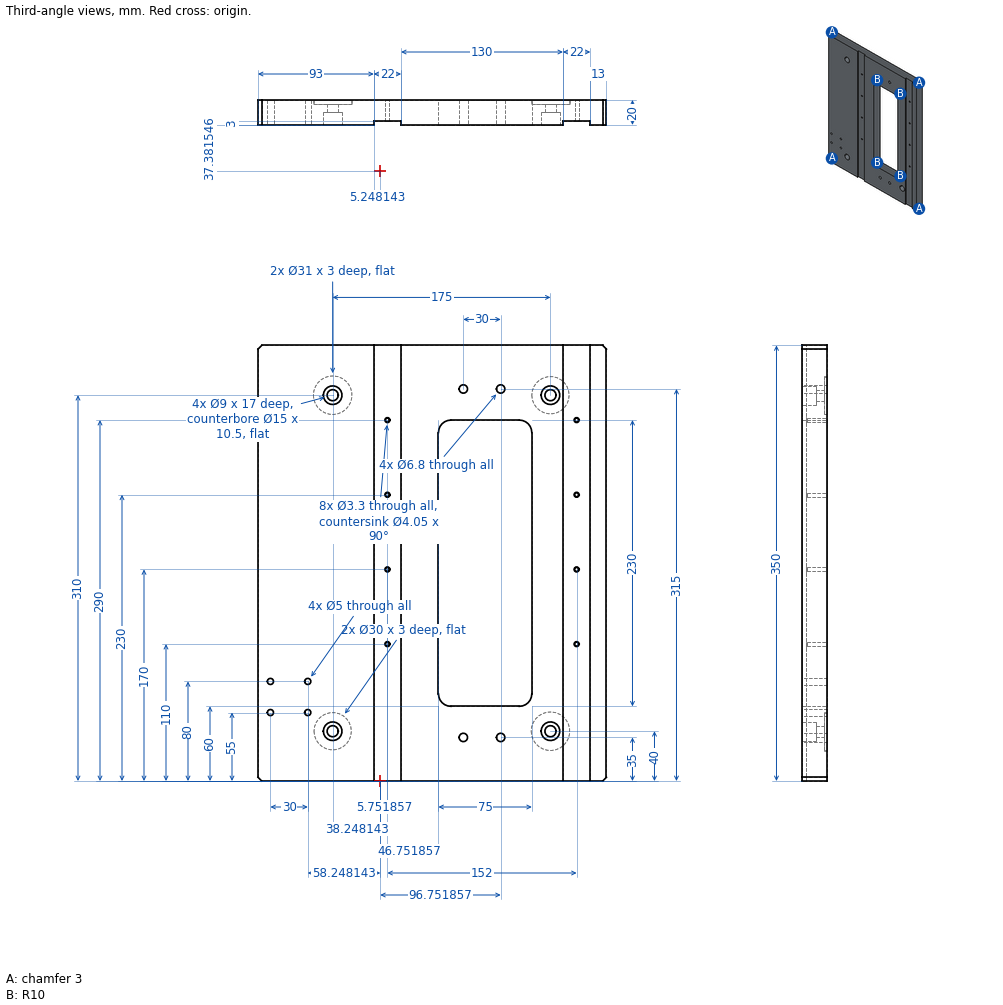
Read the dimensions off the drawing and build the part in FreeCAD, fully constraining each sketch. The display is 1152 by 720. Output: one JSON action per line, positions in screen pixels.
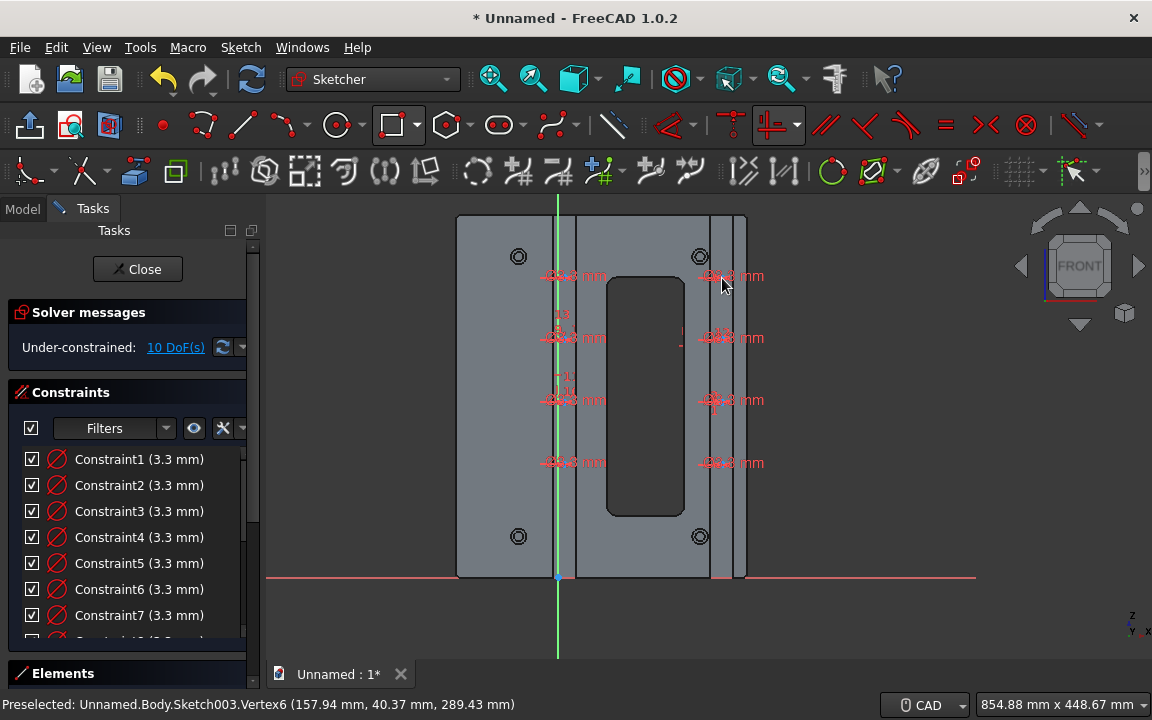
{"action": "left_click", "coordinate": [564, 278]}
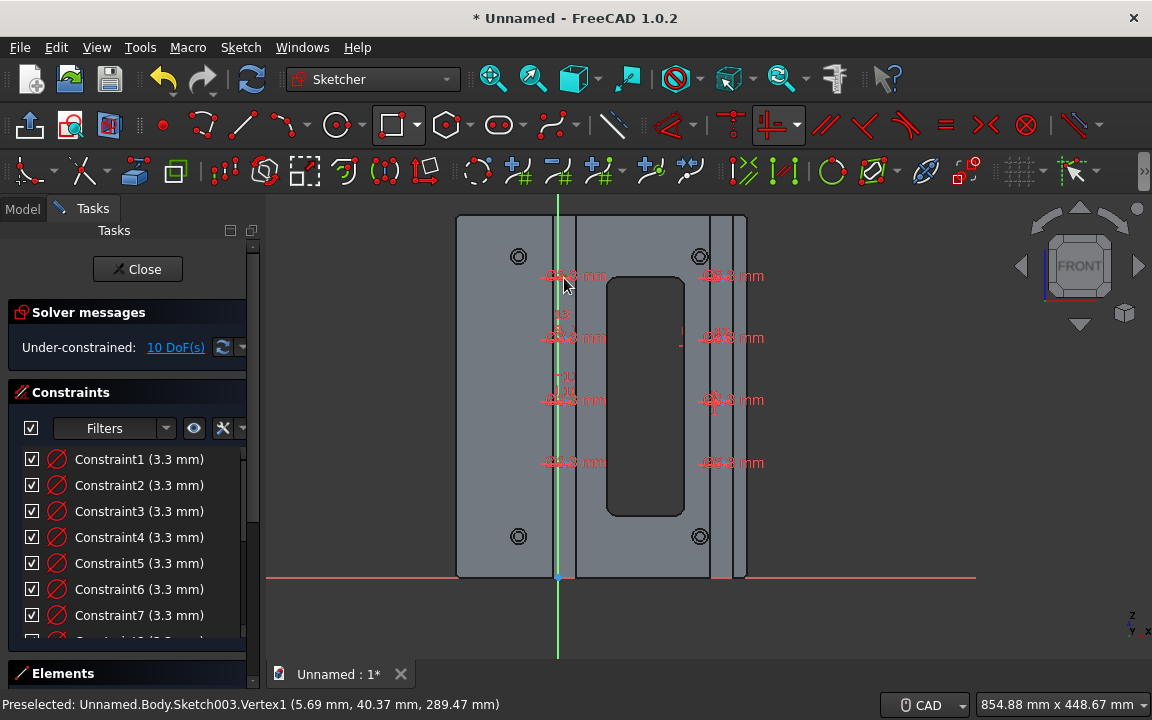
{"action": "left_click", "coordinate": [722, 278]}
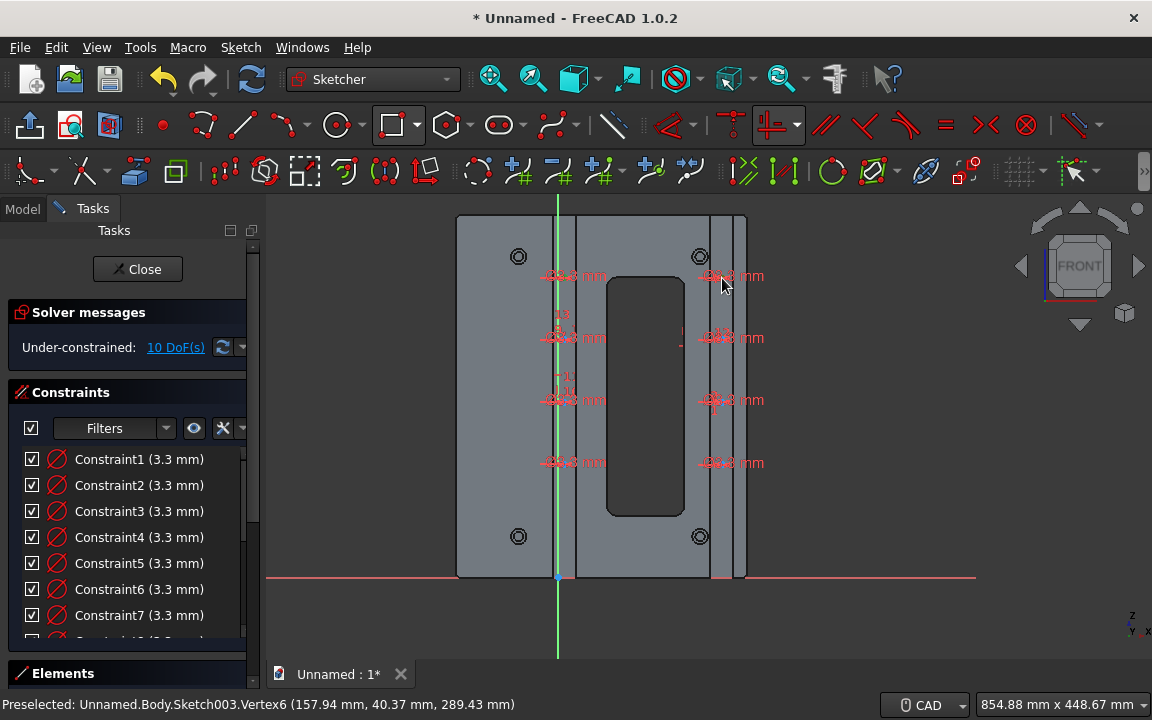
{"action": "left_click", "coordinate": [800, 126]}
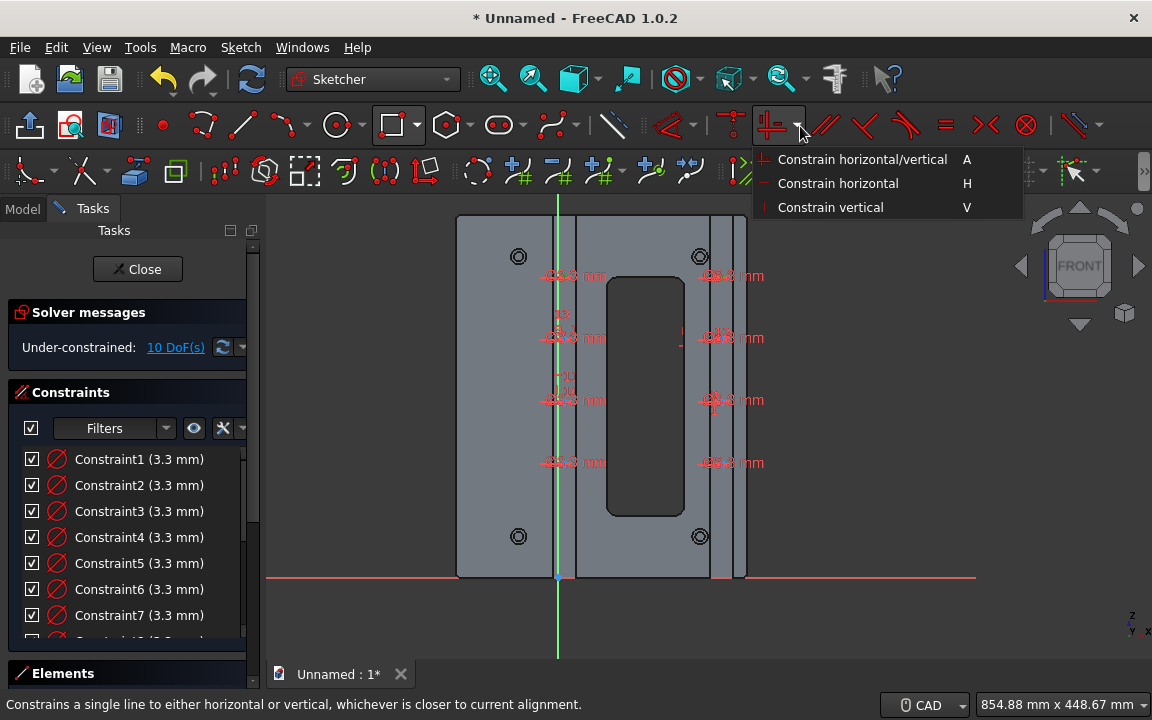
{"action": "left_click", "coordinate": [888, 183]}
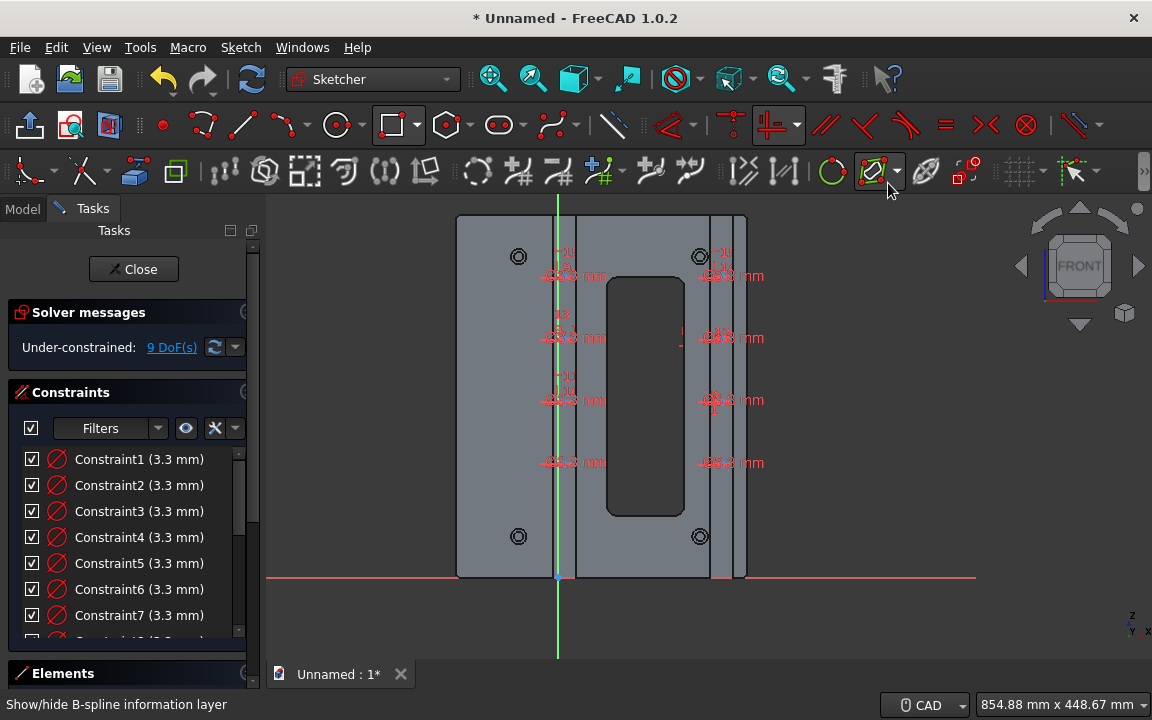
{"action": "left_click", "coordinate": [564, 402]}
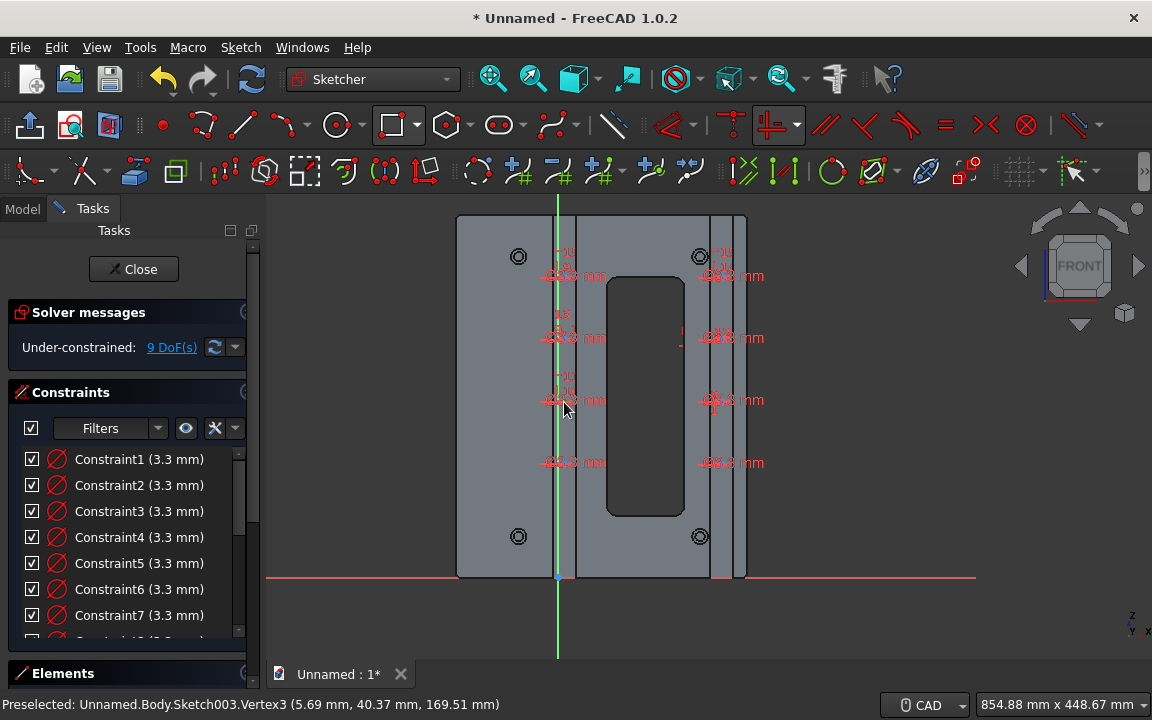
{"action": "left_click", "coordinate": [564, 464]}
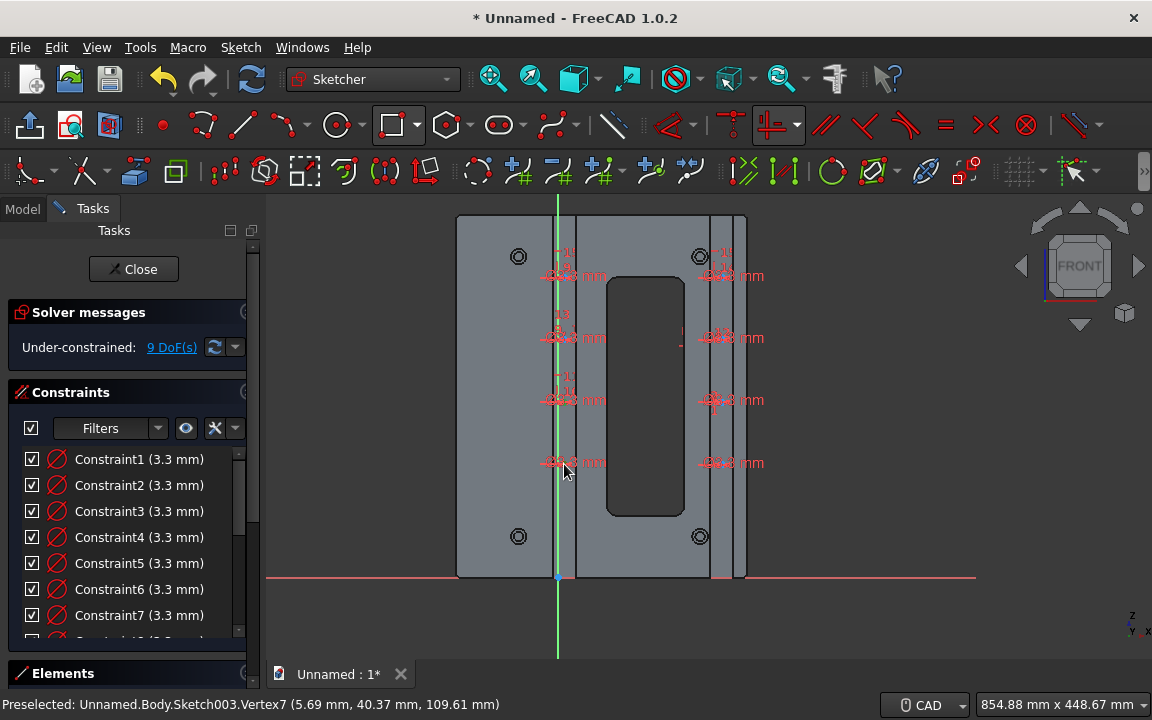
{"action": "left_click", "coordinate": [800, 126]}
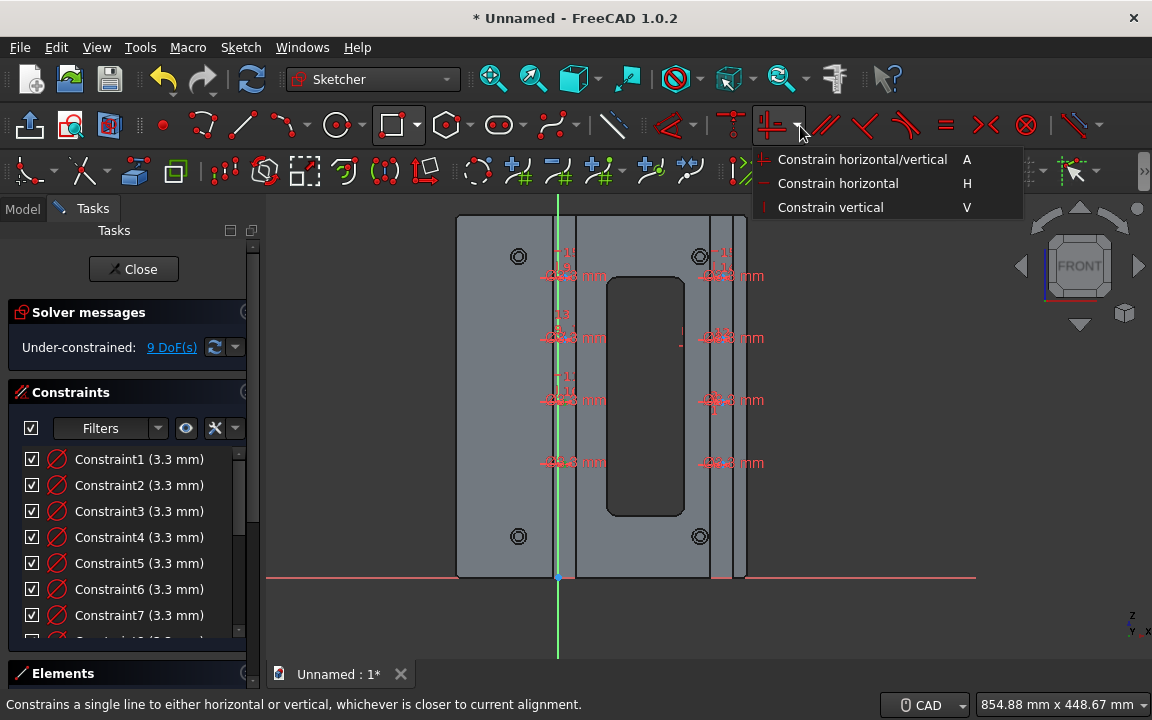
{"action": "left_click", "coordinate": [888, 207]}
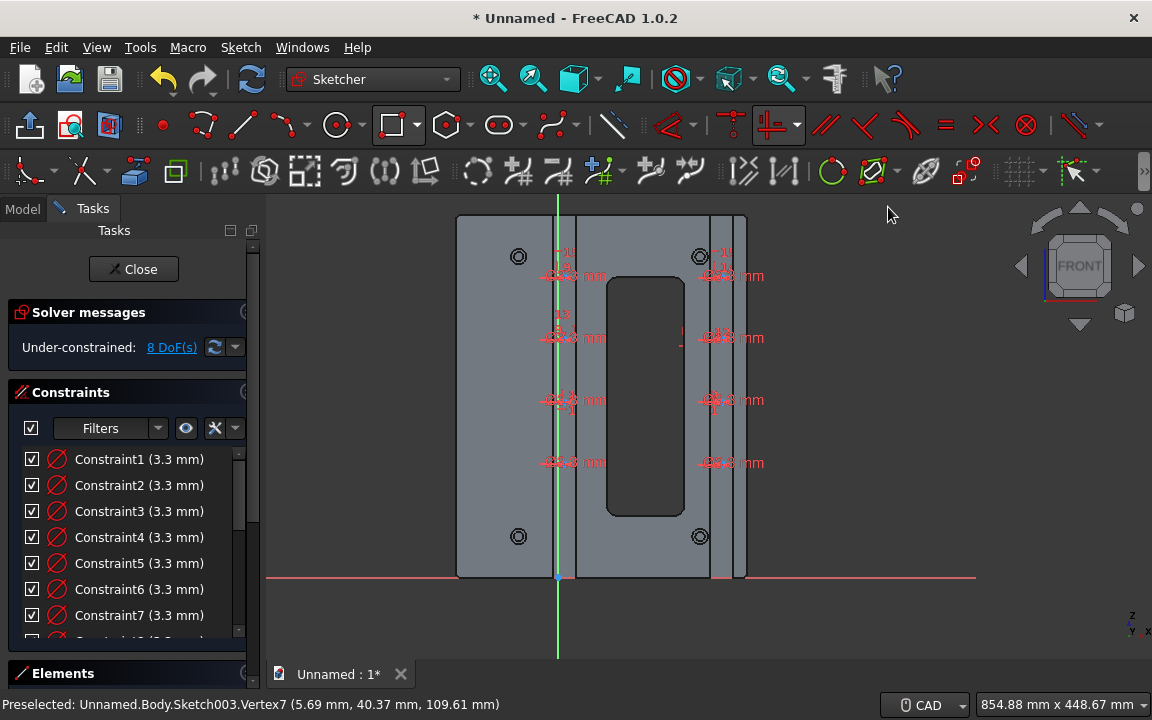
{"action": "left_click", "coordinate": [722, 402]}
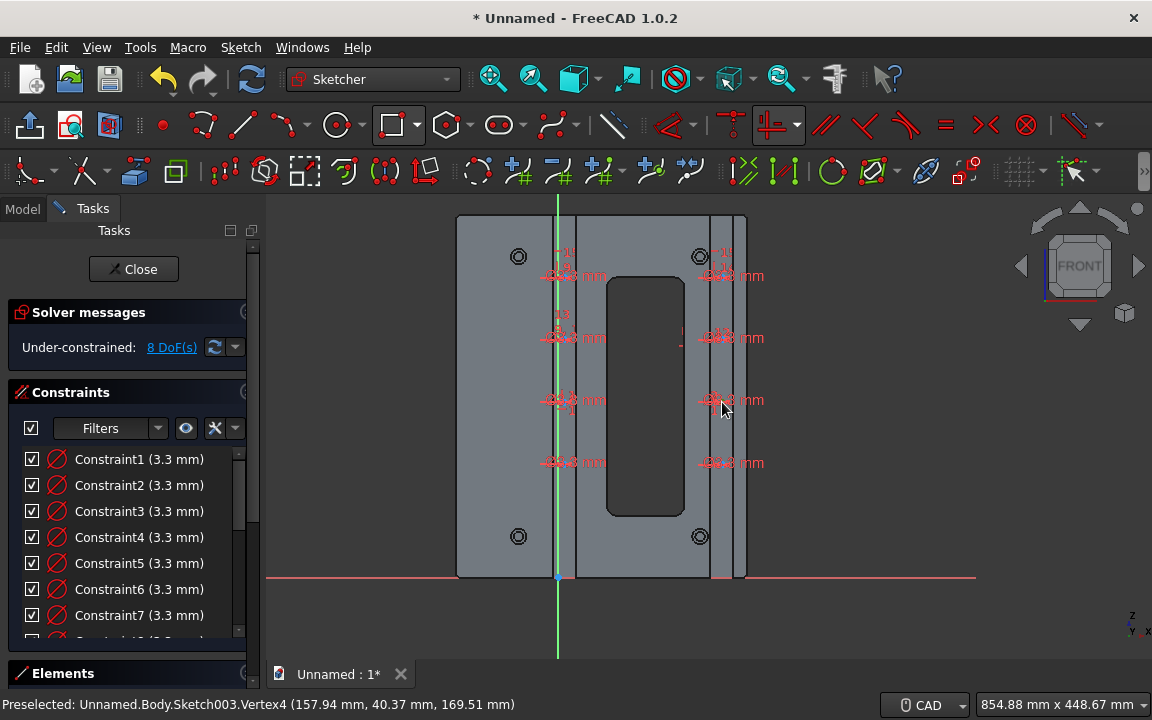
{"action": "left_click", "coordinate": [722, 465]}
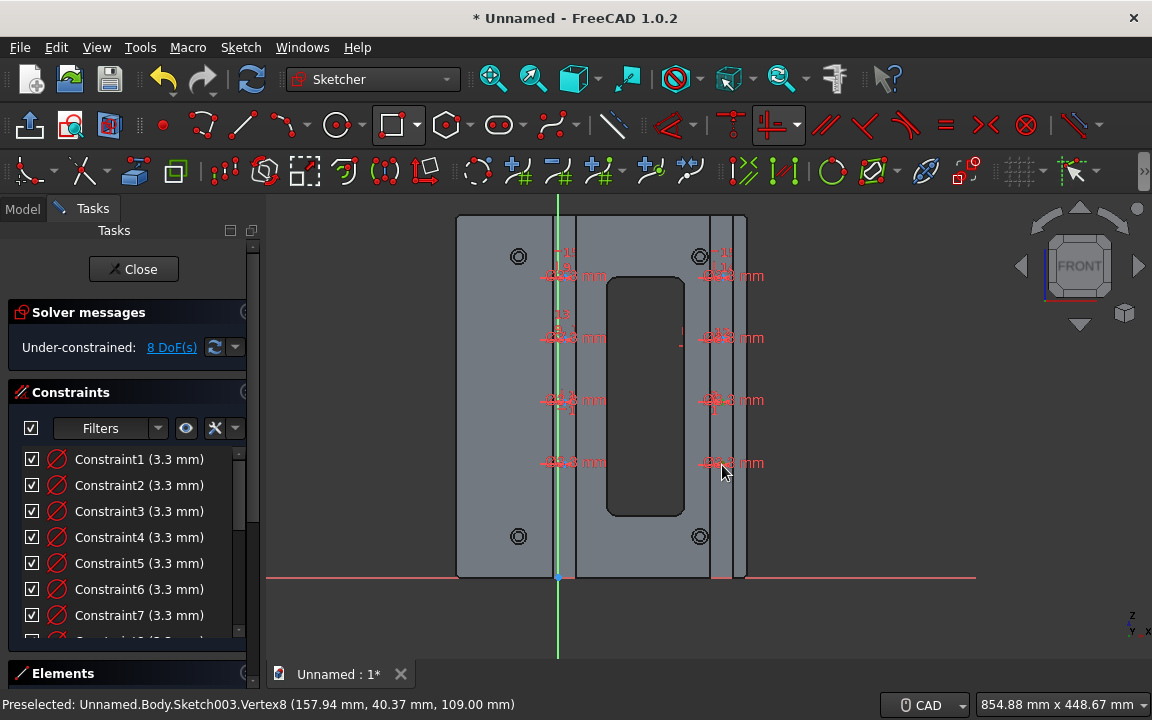
{"action": "left_click", "coordinate": [800, 126]}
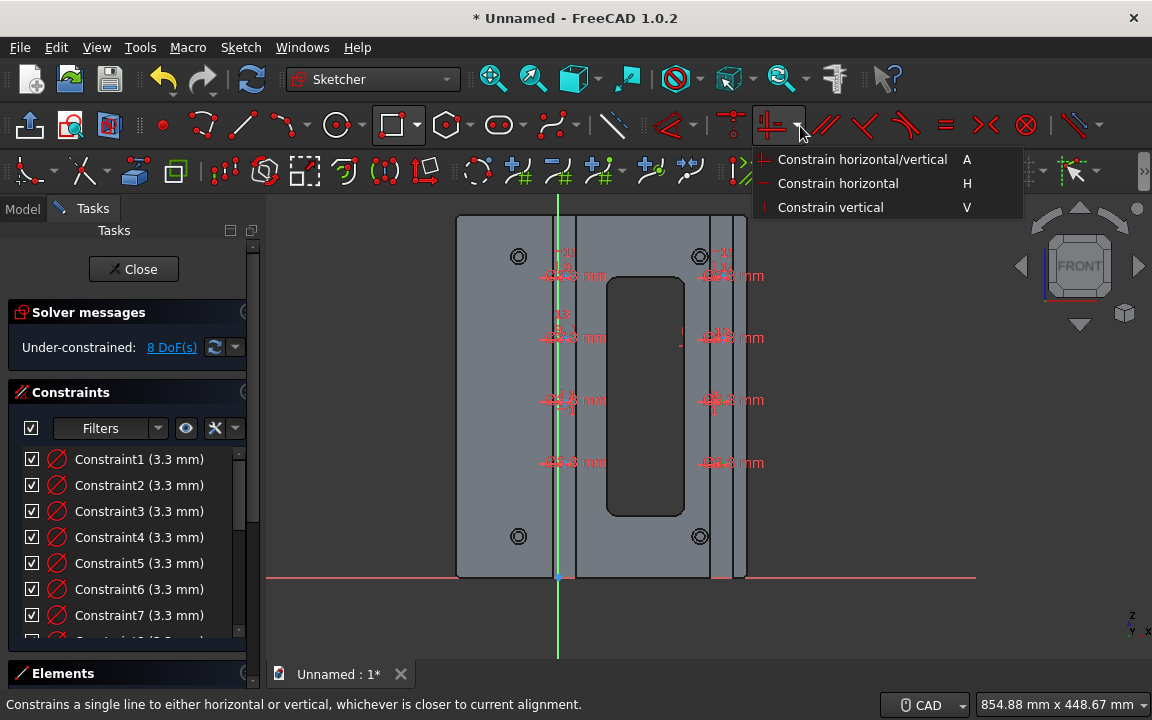
{"action": "left_click", "coordinate": [888, 207]}